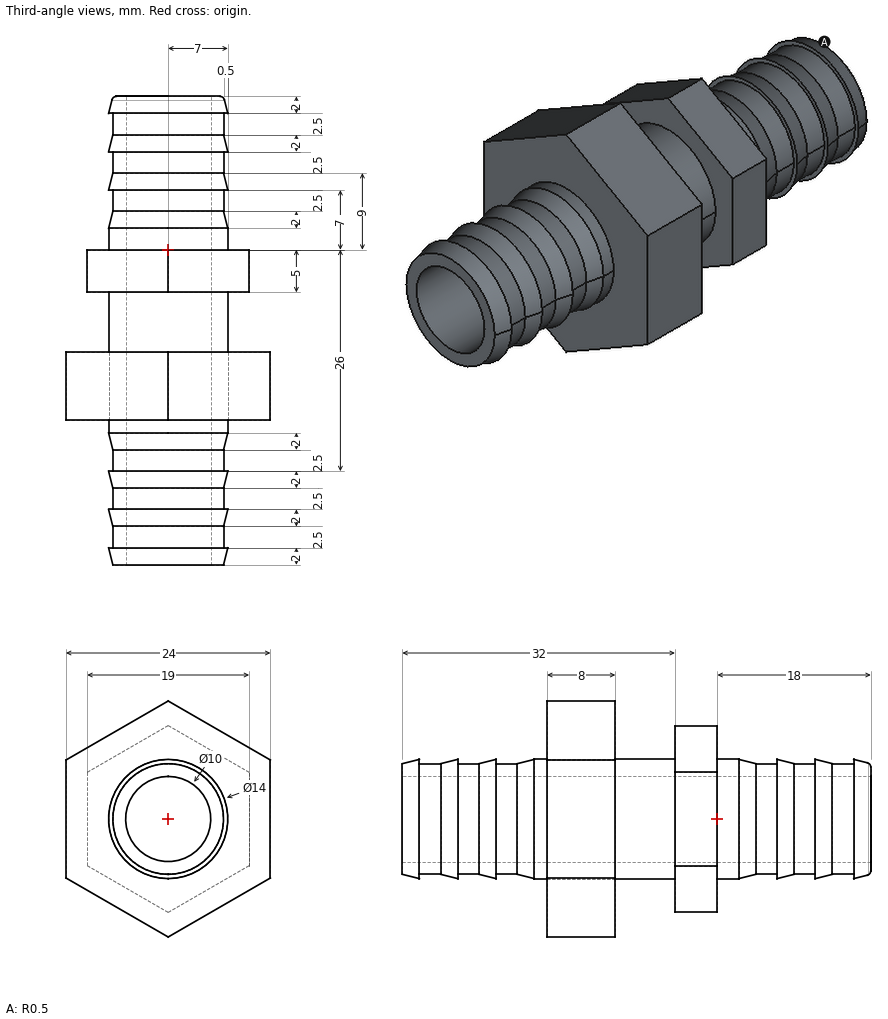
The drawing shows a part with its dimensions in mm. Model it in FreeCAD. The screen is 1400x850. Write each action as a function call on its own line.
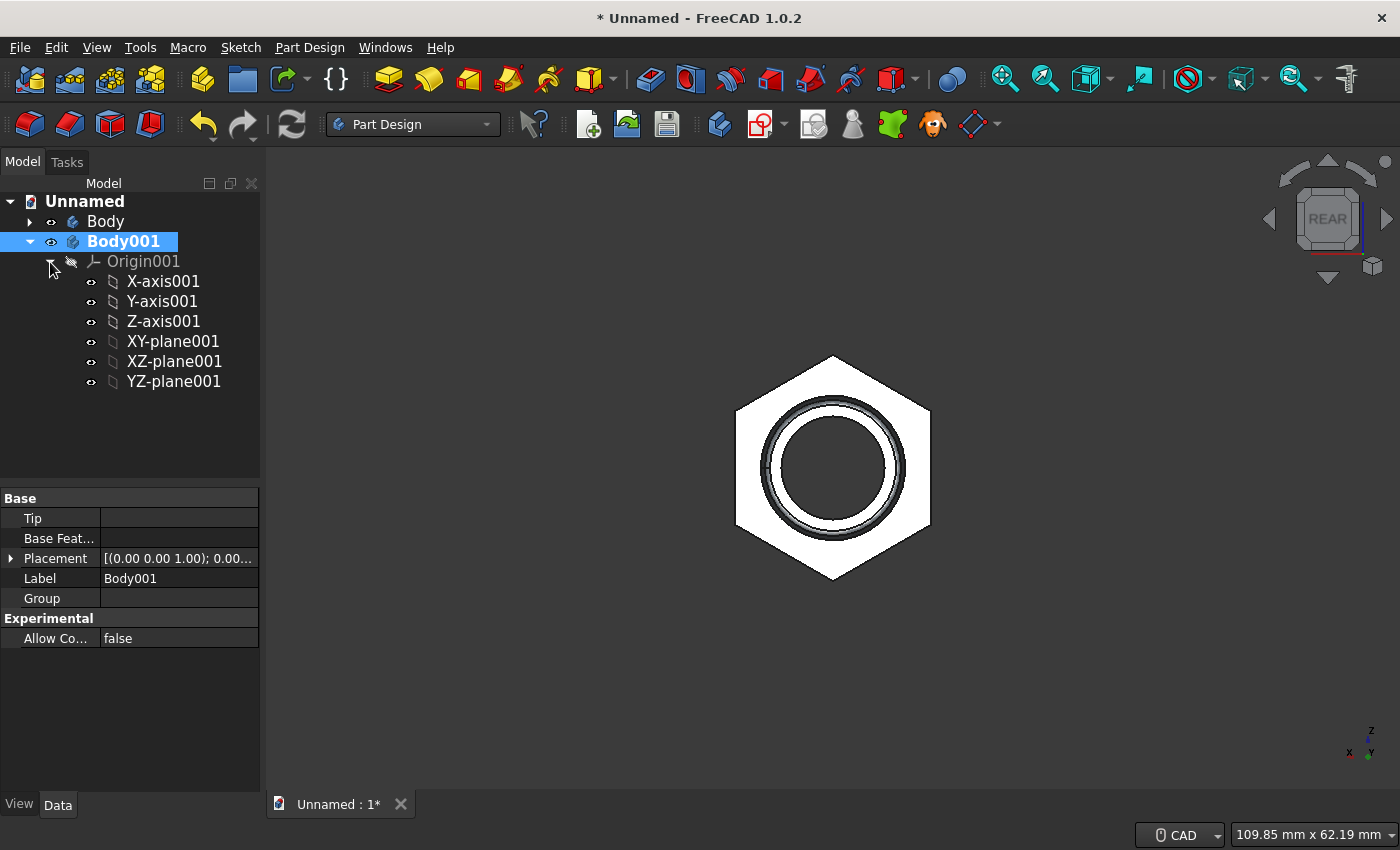
click(136, 362)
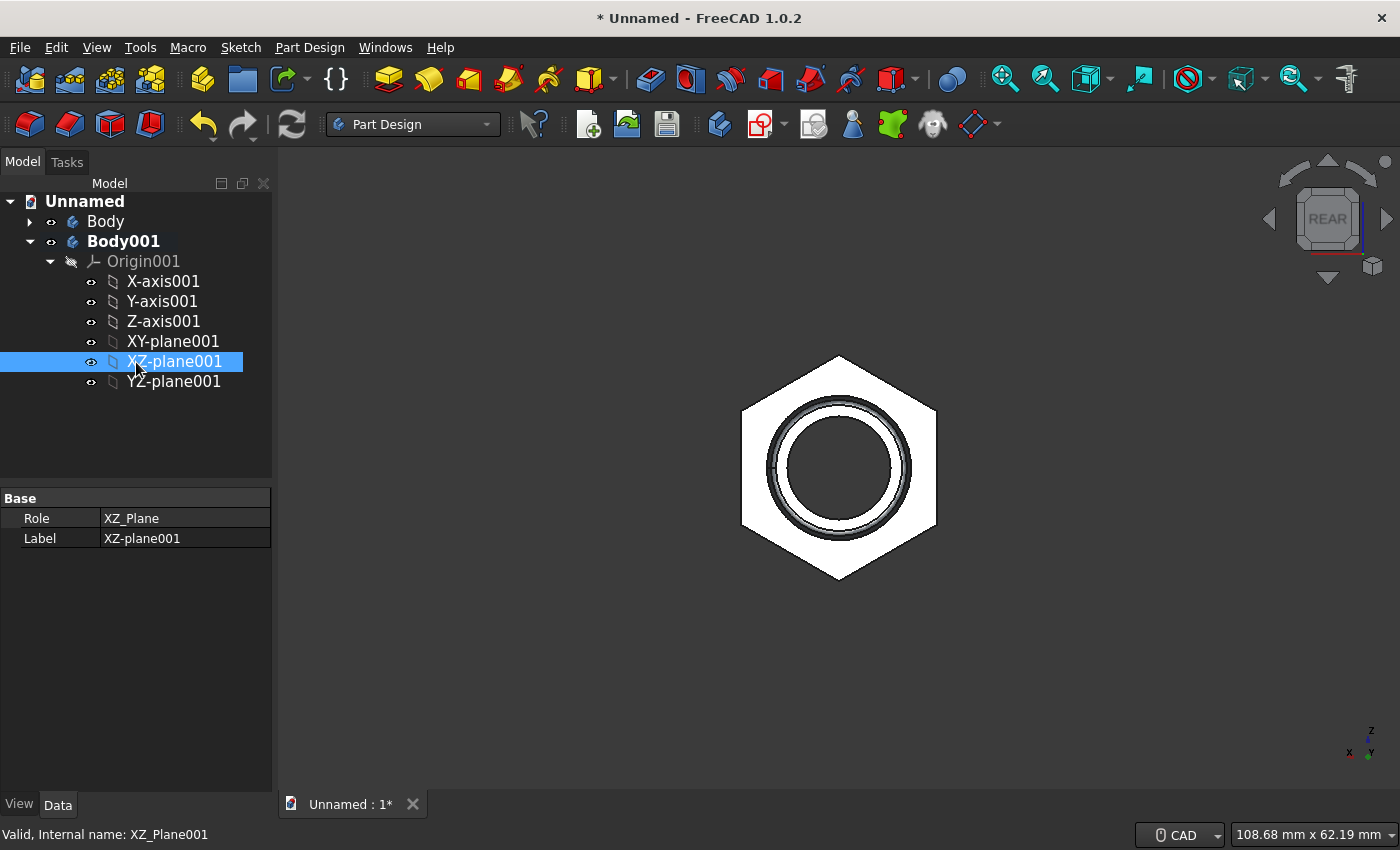
click(974, 124)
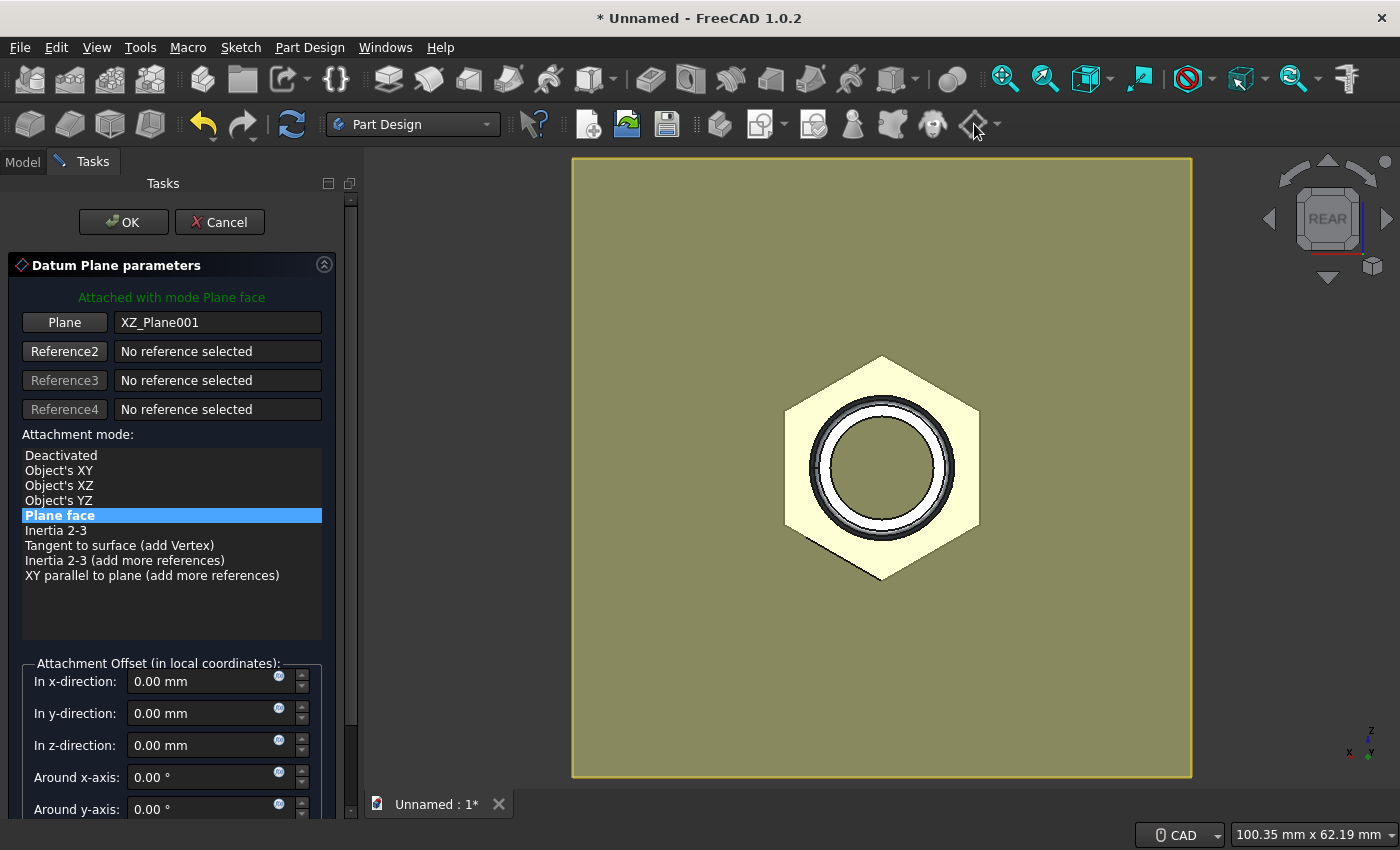
triple_click(210, 745)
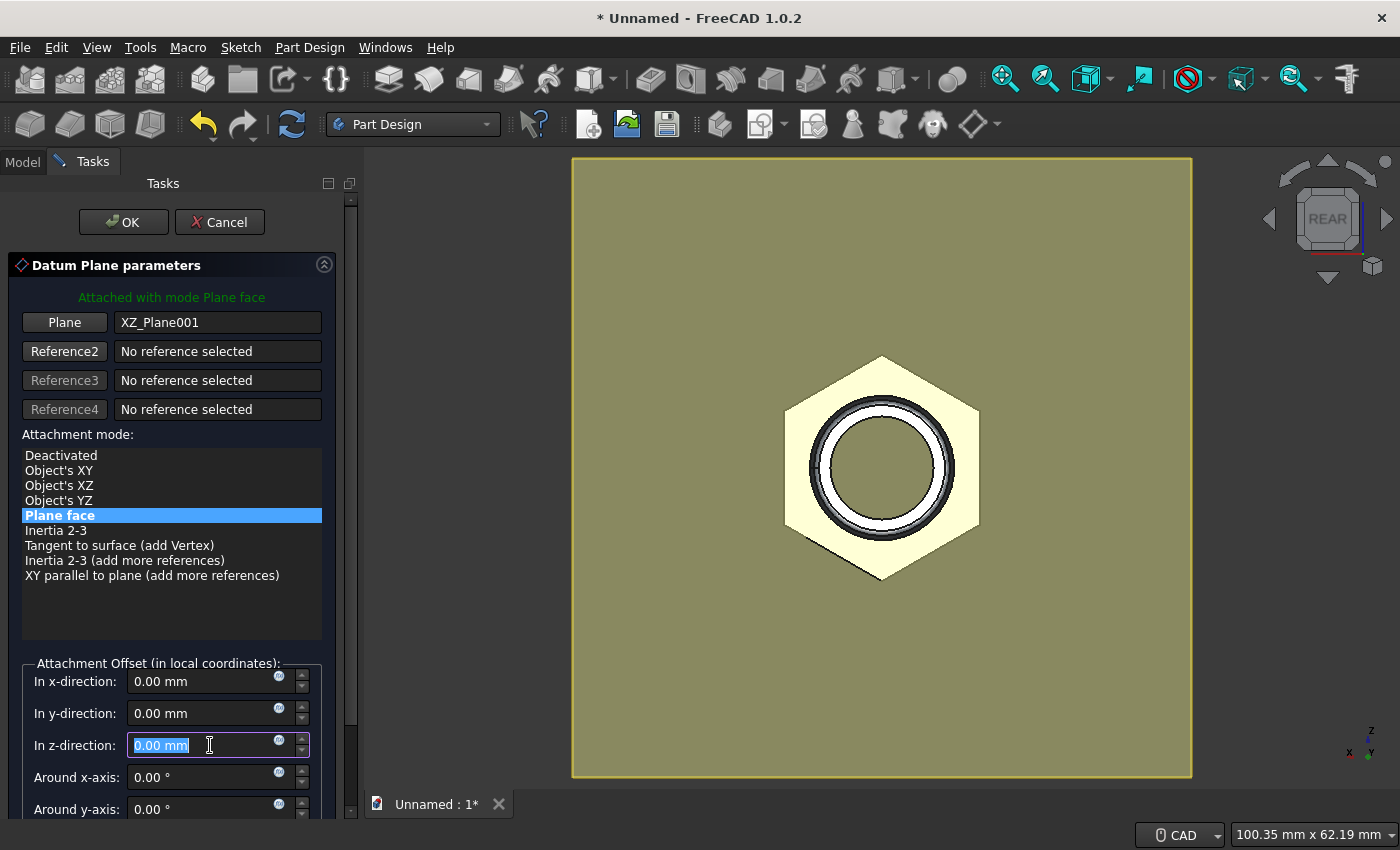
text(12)
key(Tab)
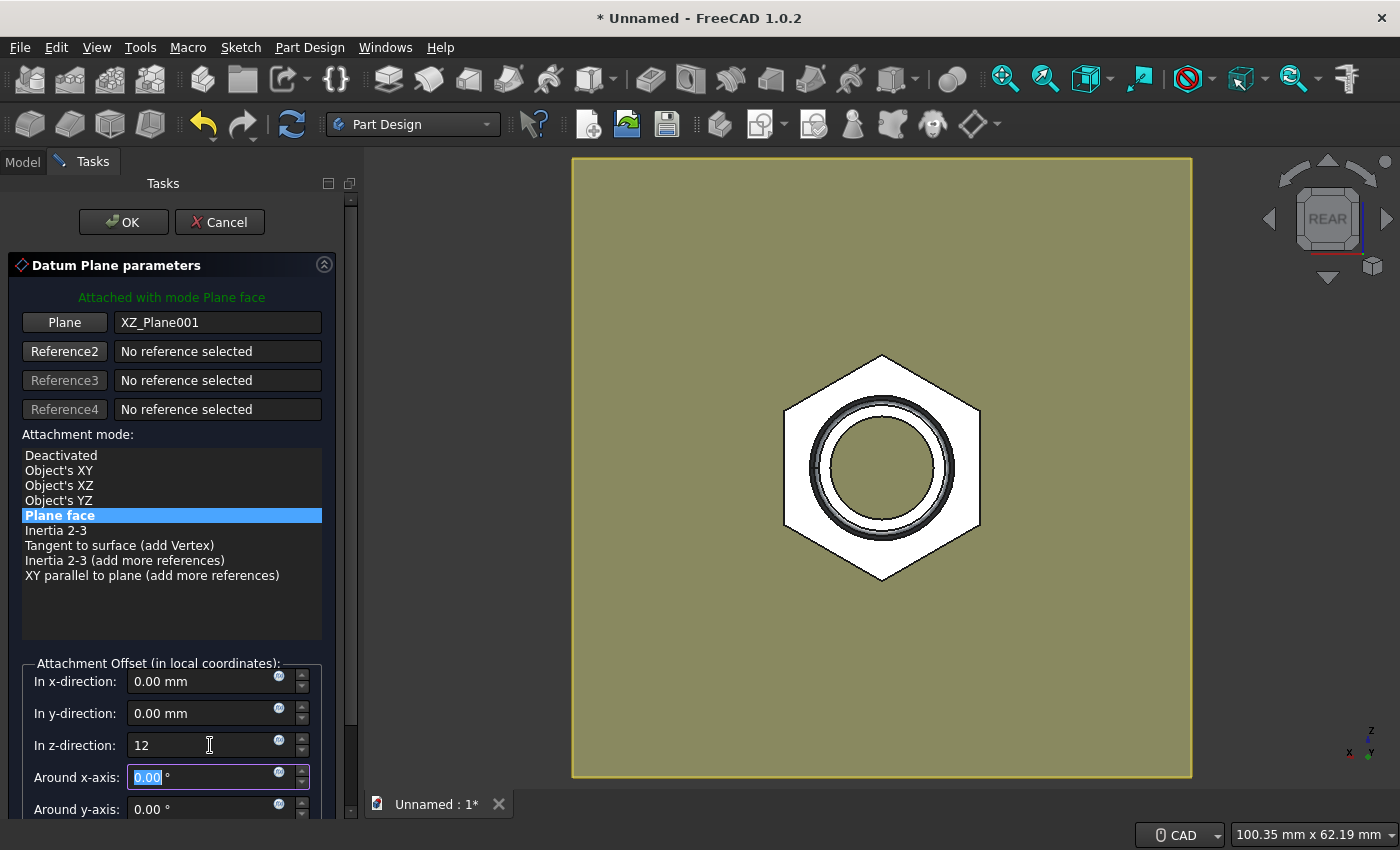
click(124, 222)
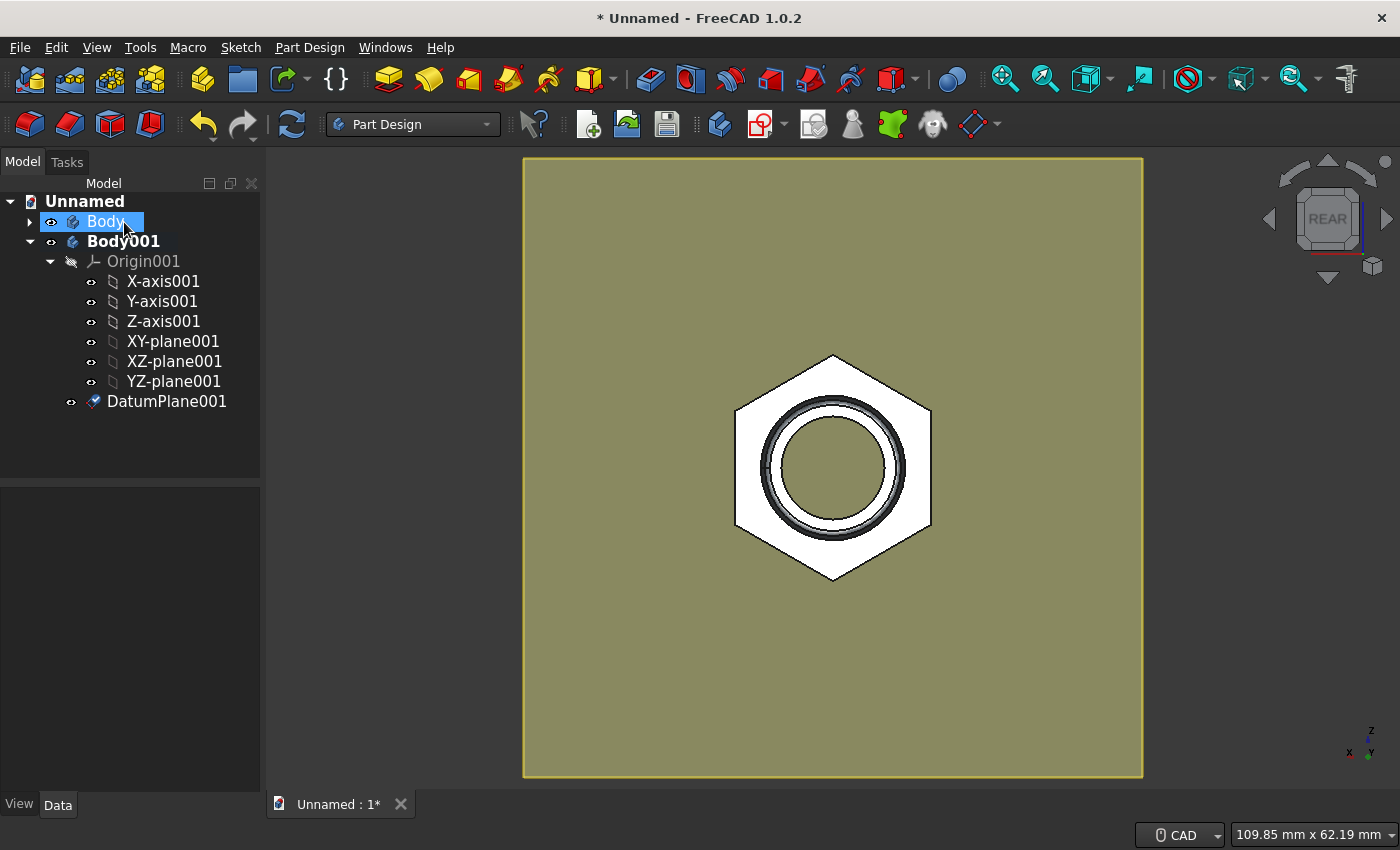
click(116, 402)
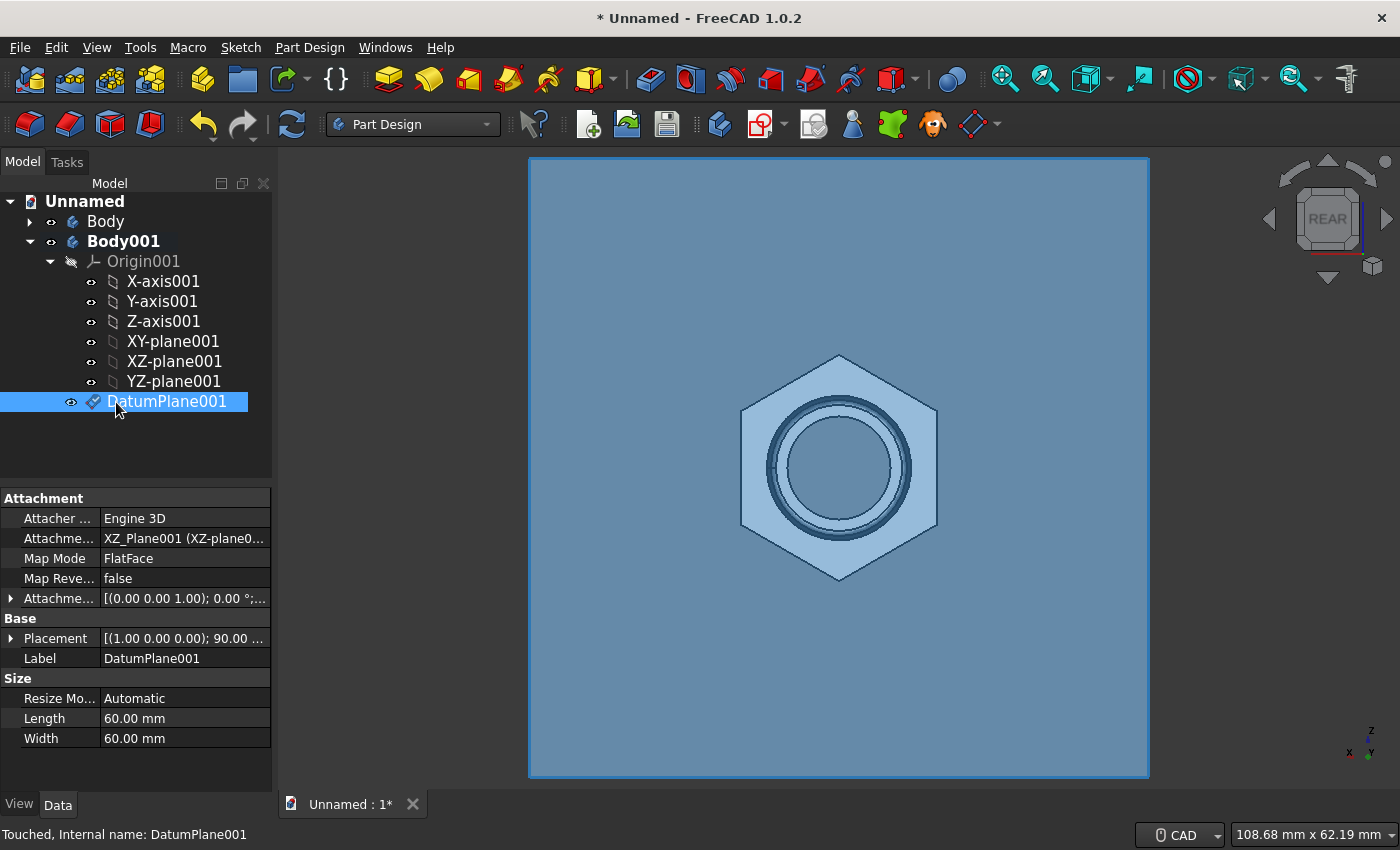
click(760, 124)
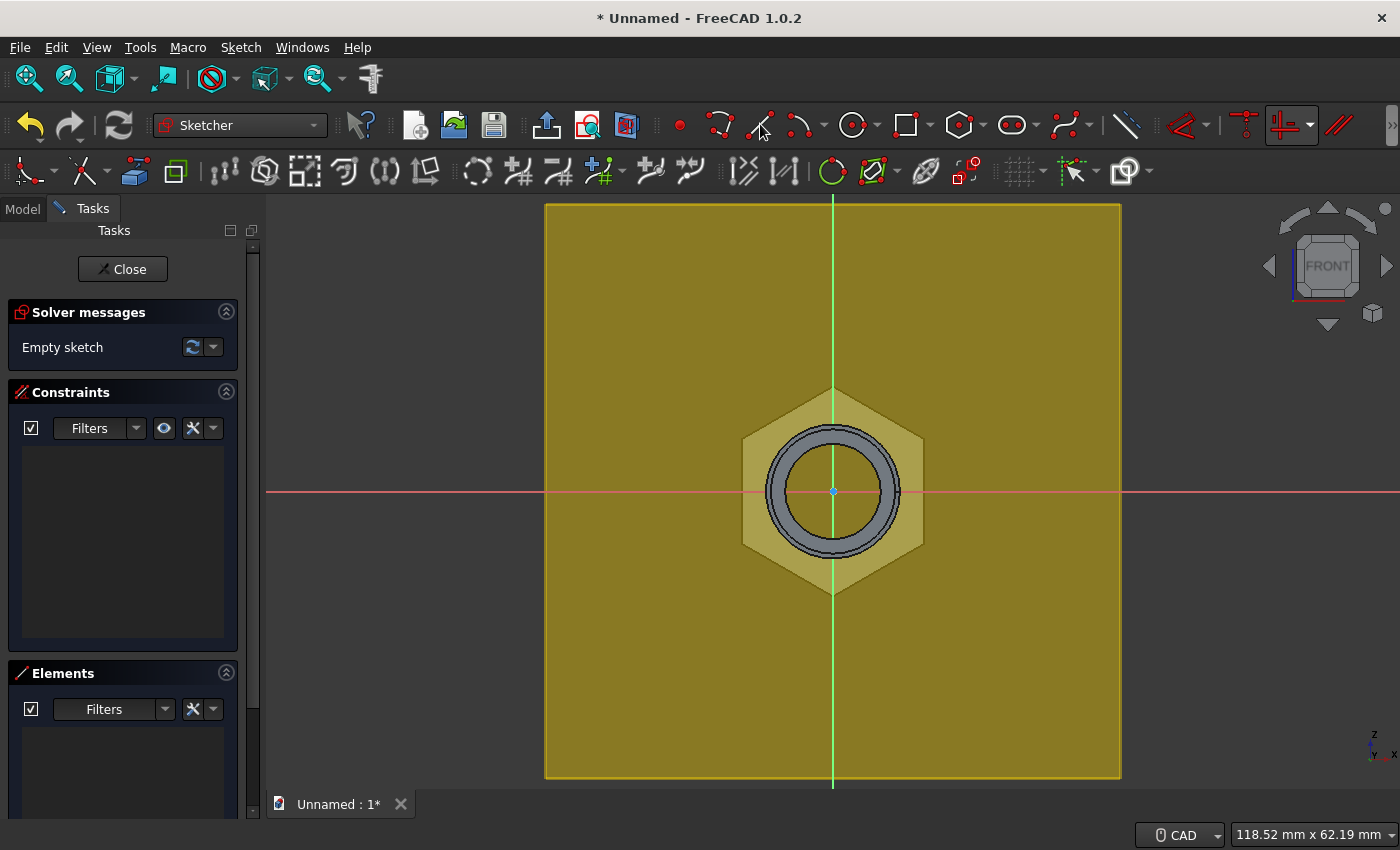
scroll(972, 491, up, 2)